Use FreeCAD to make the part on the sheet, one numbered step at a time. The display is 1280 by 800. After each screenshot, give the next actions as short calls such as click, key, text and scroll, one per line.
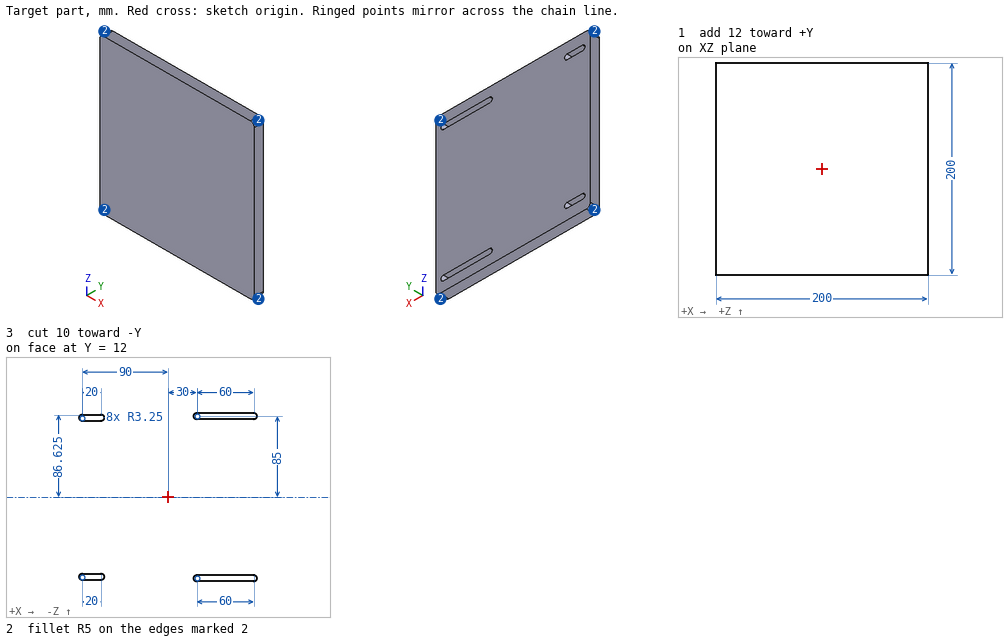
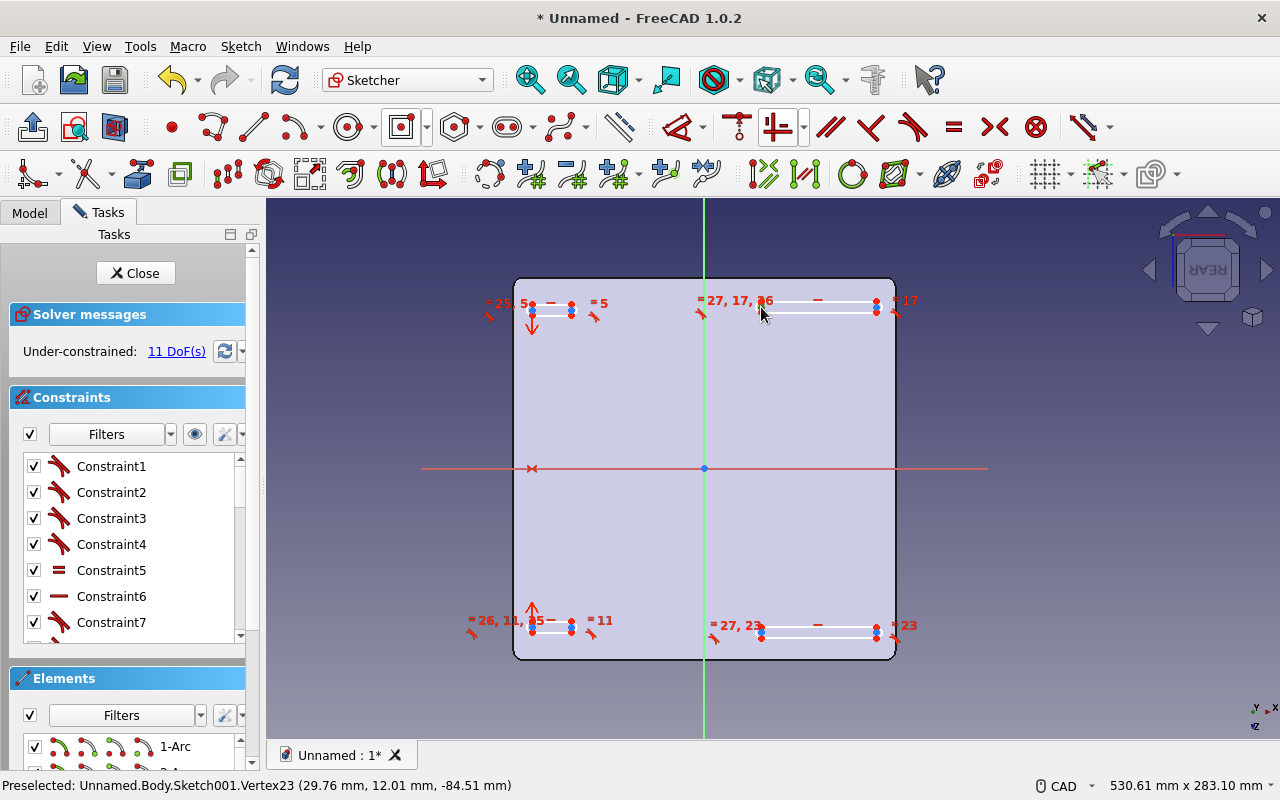
scroll(761, 633, up, 5)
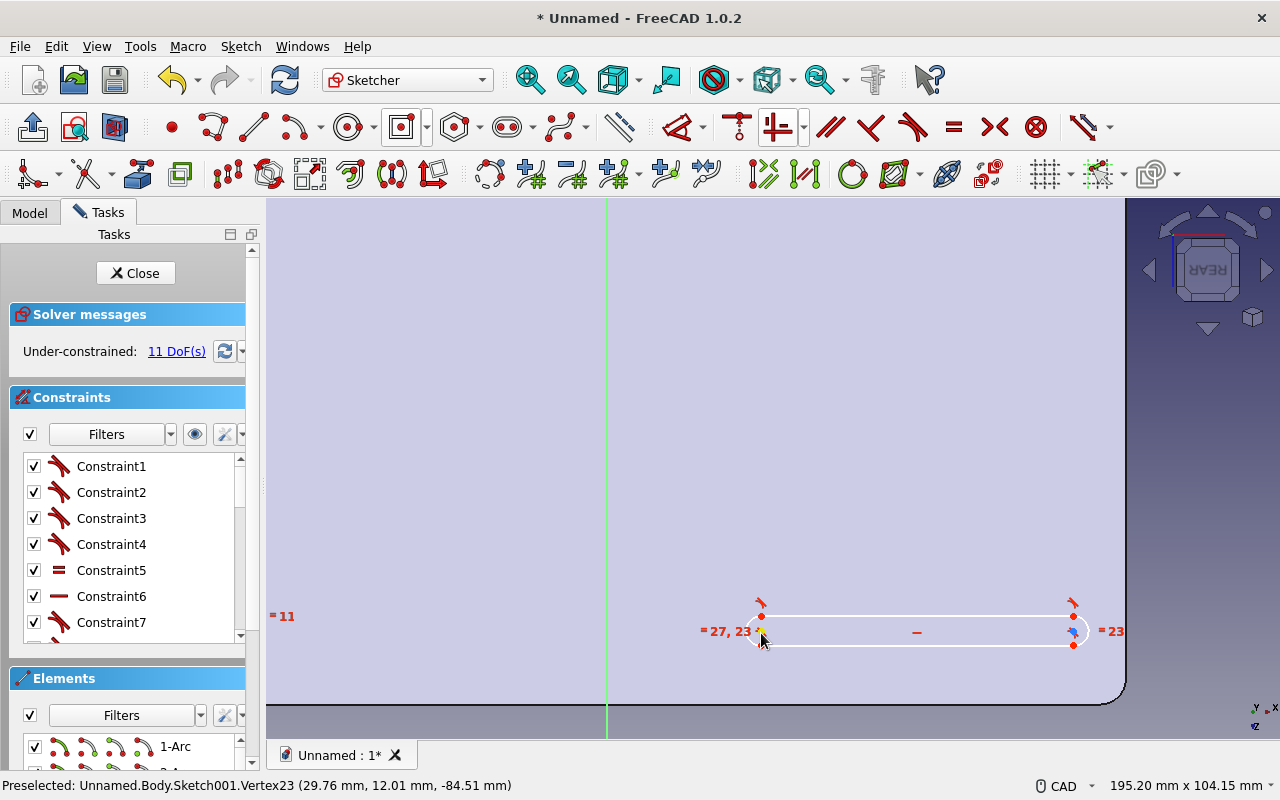
click(761, 631)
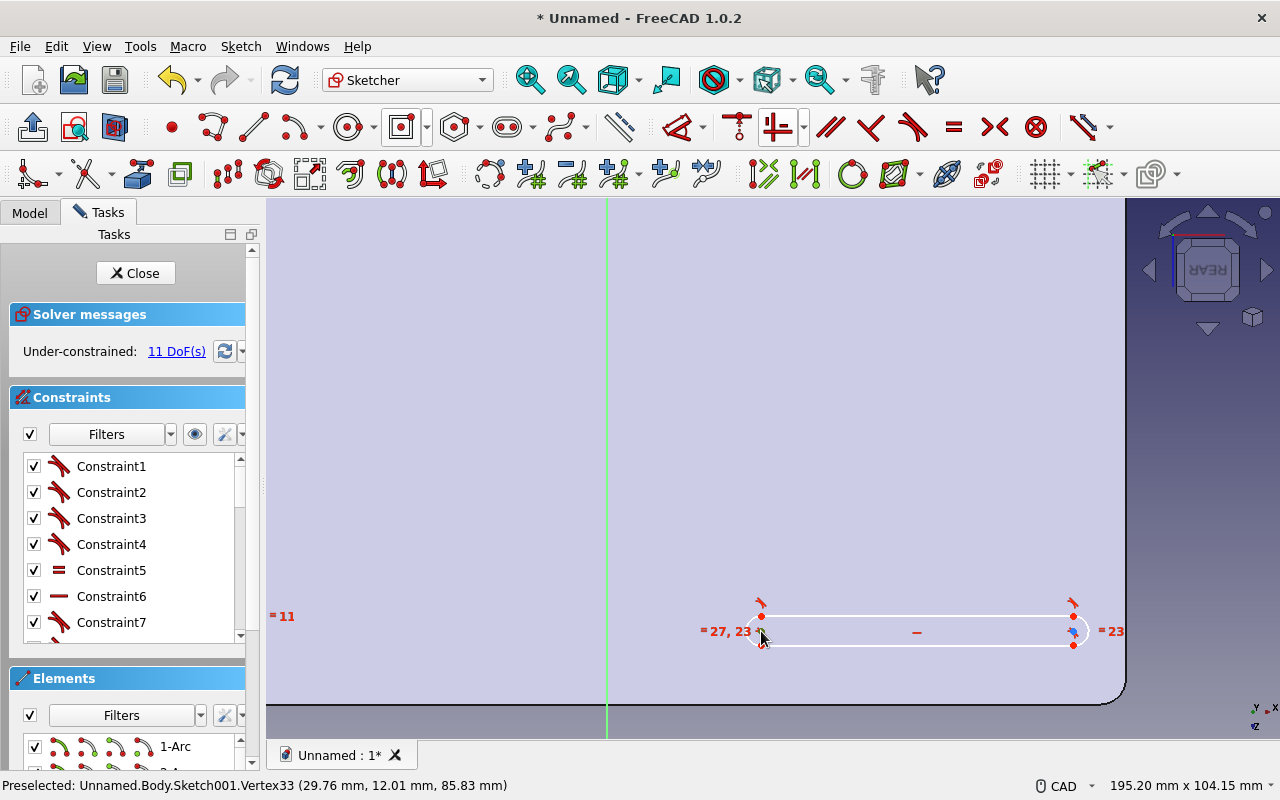
scroll(761, 633, down, 5)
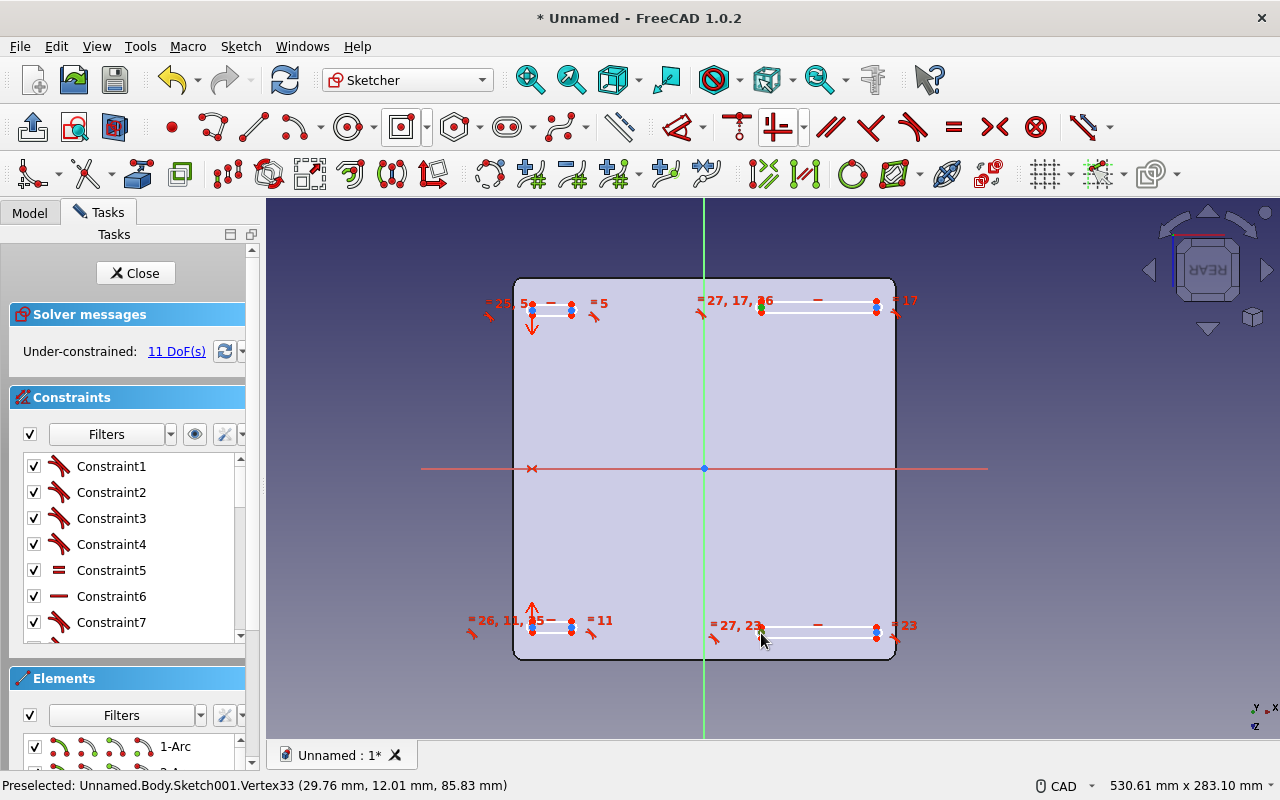
click(470, 469)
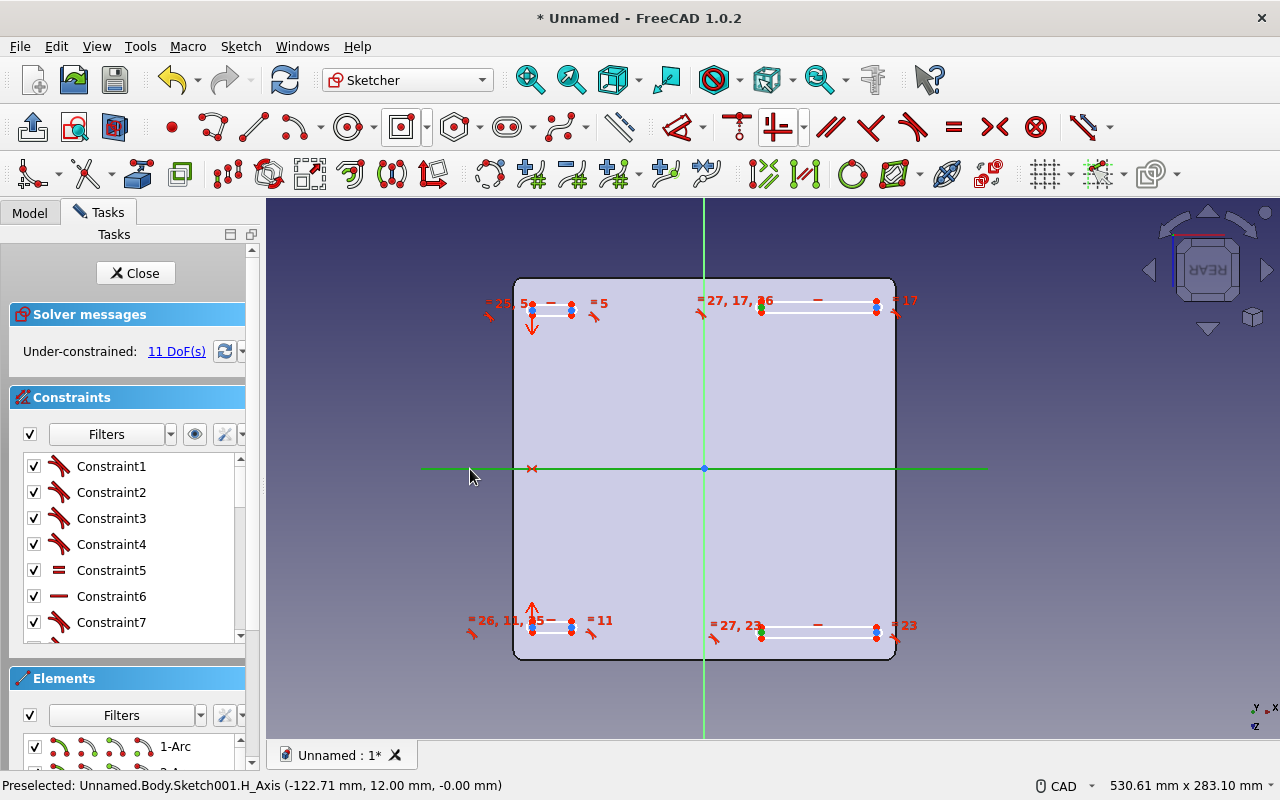
click(995, 128)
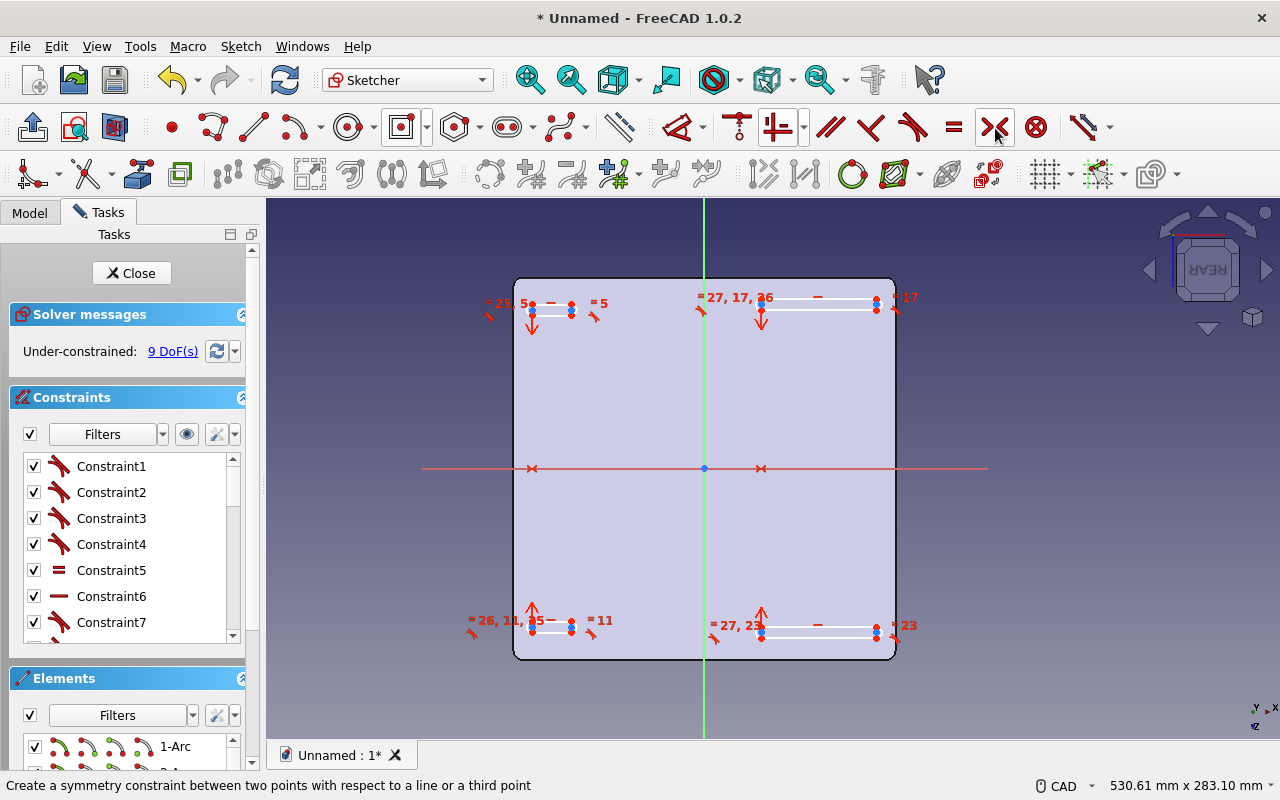
click(676, 128)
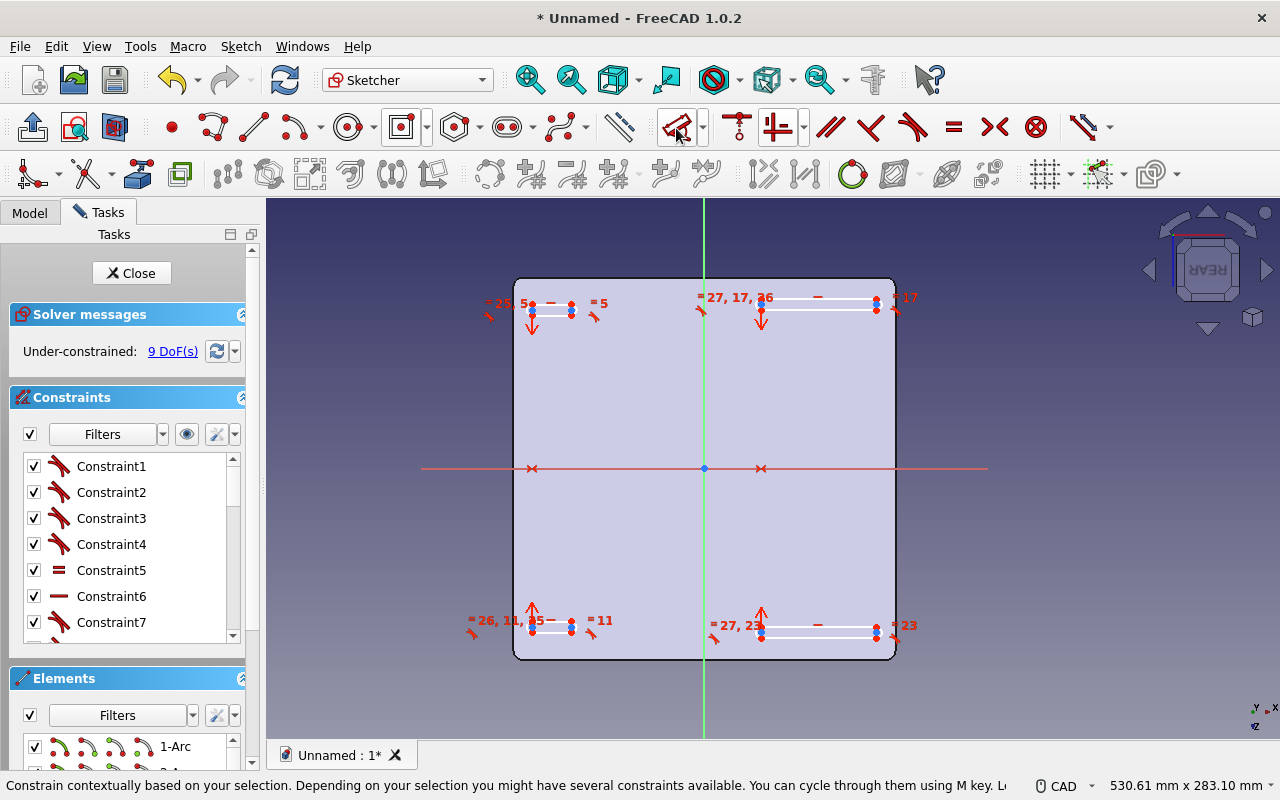
scroll(527, 310, up, 10)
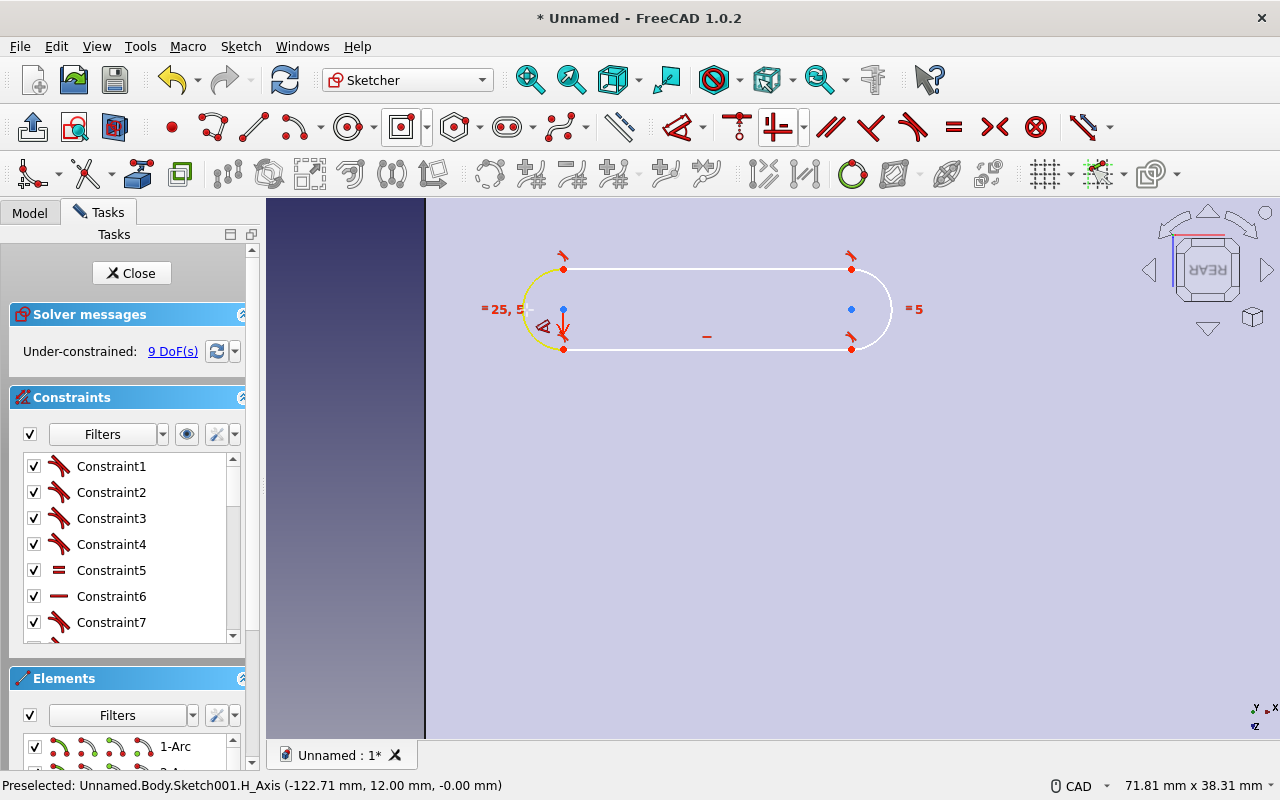
click(523, 310)
click(491, 310)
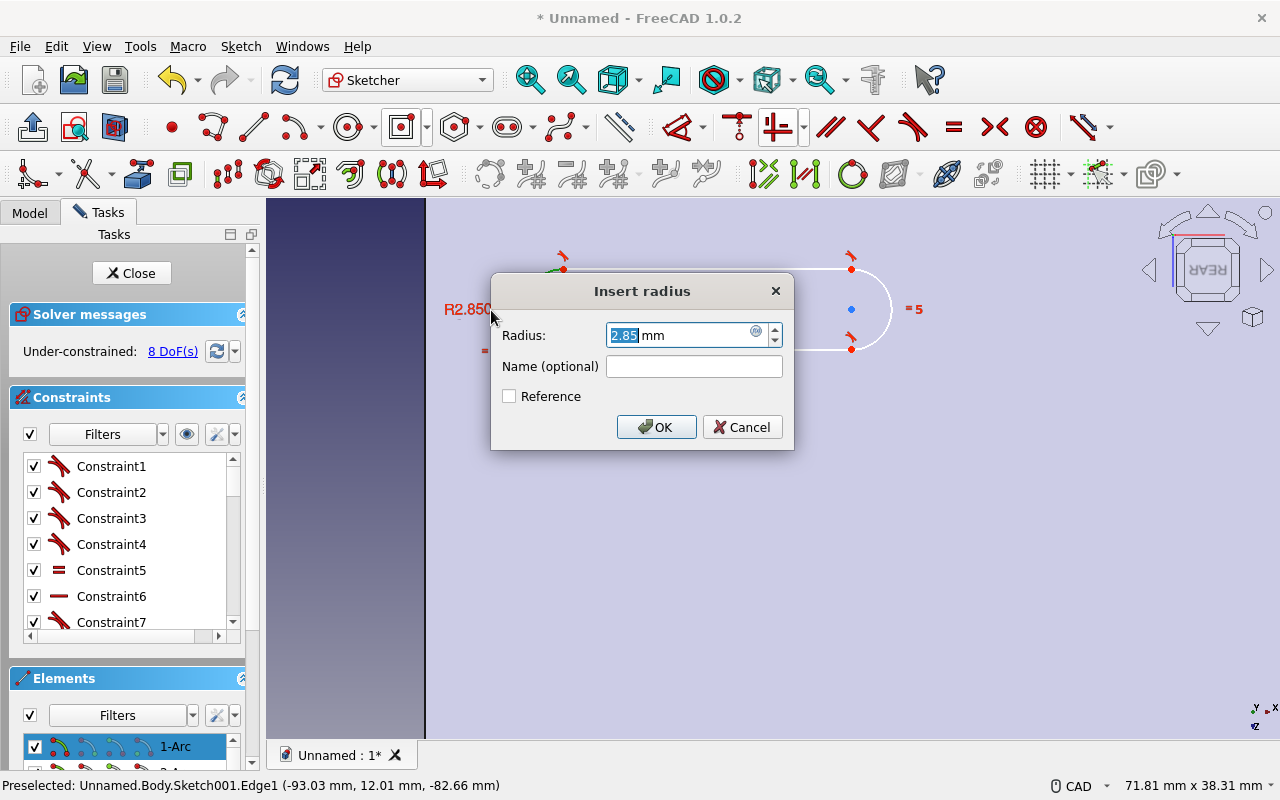
text(3.25)
key(Return)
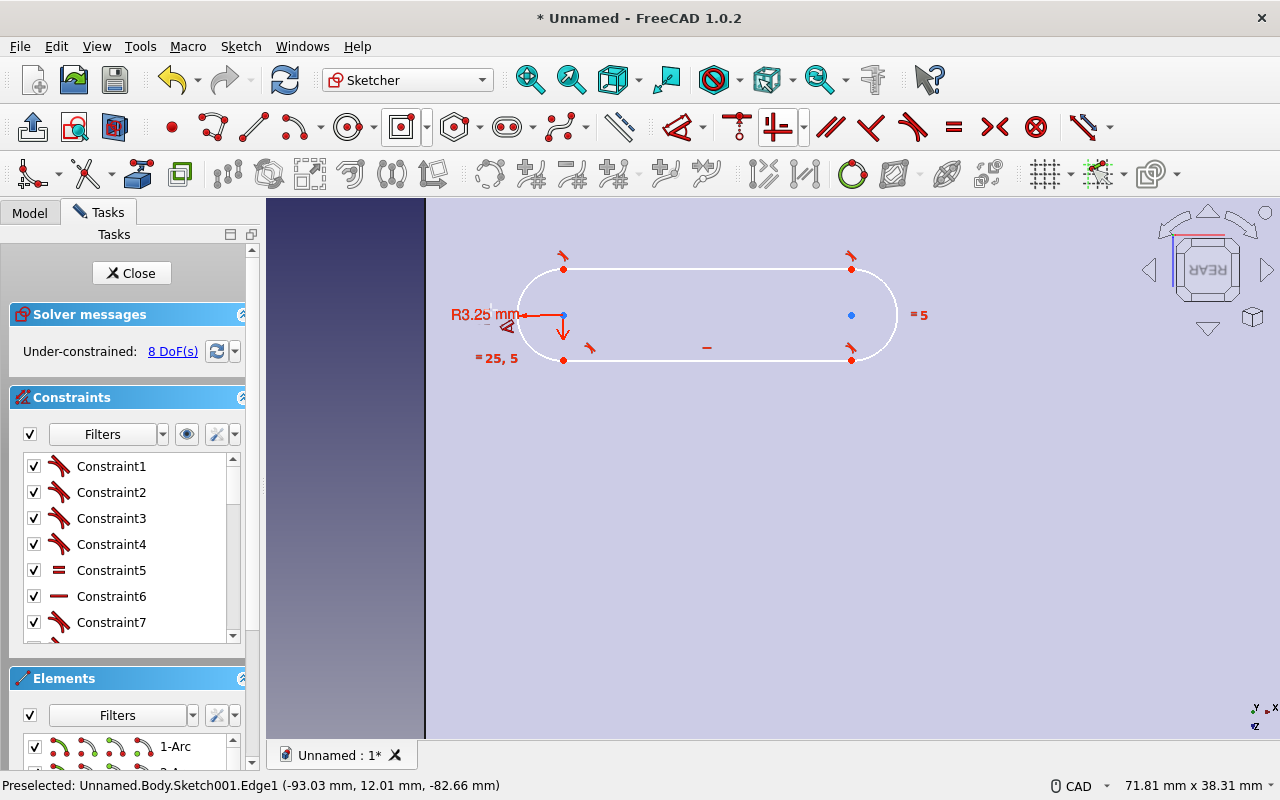
scroll(527, 310, down, 10)